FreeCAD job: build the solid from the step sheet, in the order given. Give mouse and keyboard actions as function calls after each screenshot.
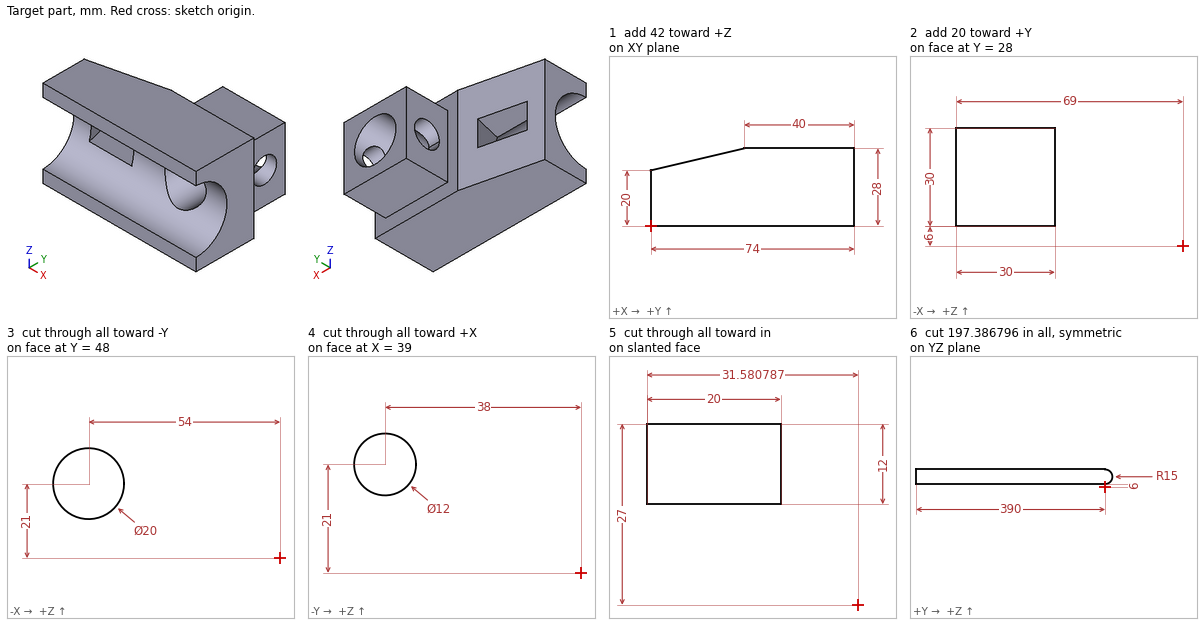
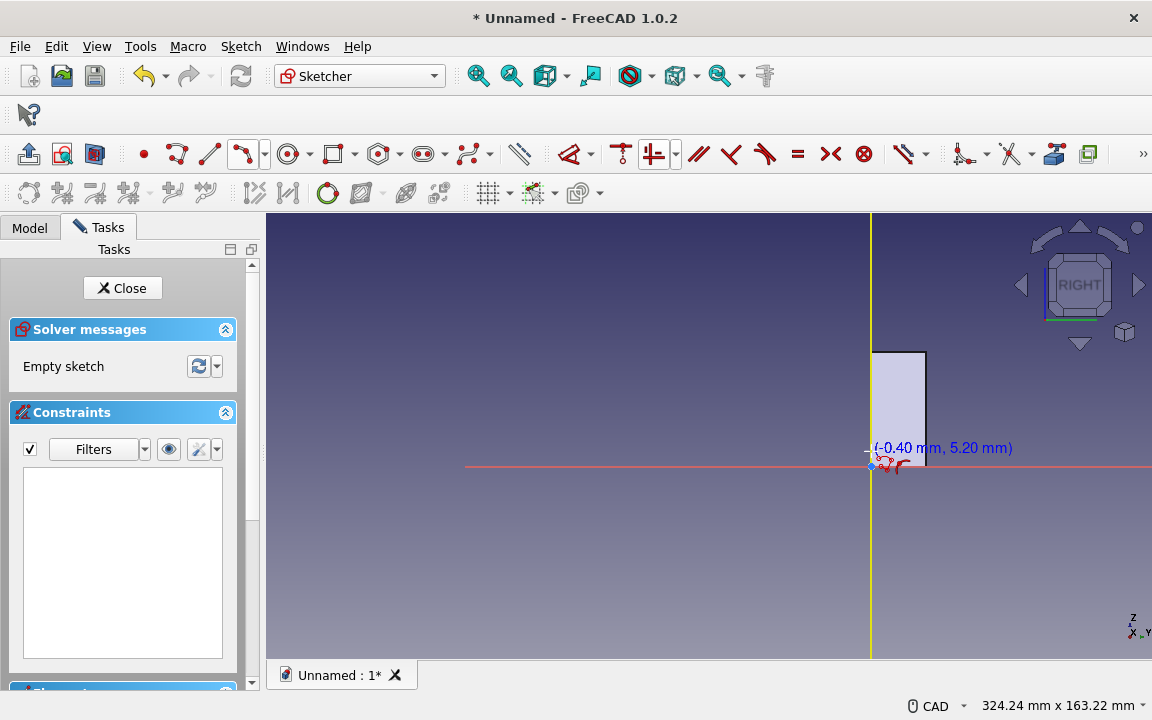
click(871, 450)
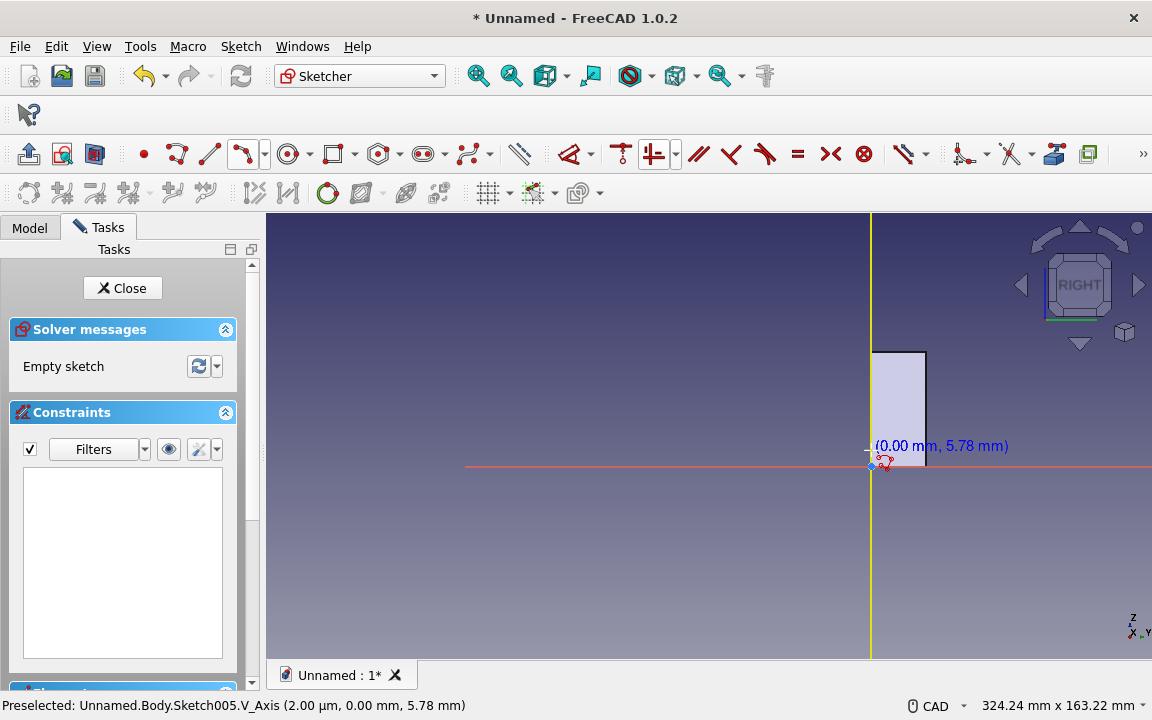
scroll(870, 451, down, 4)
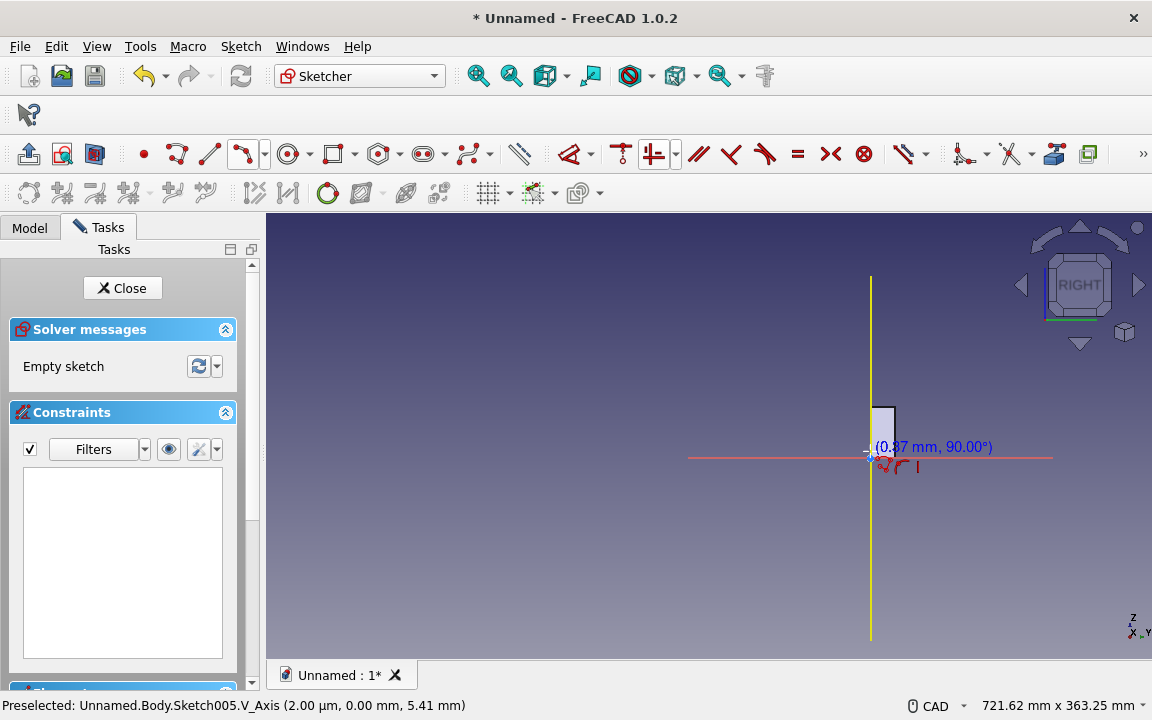
scroll(392, 451, up, 4)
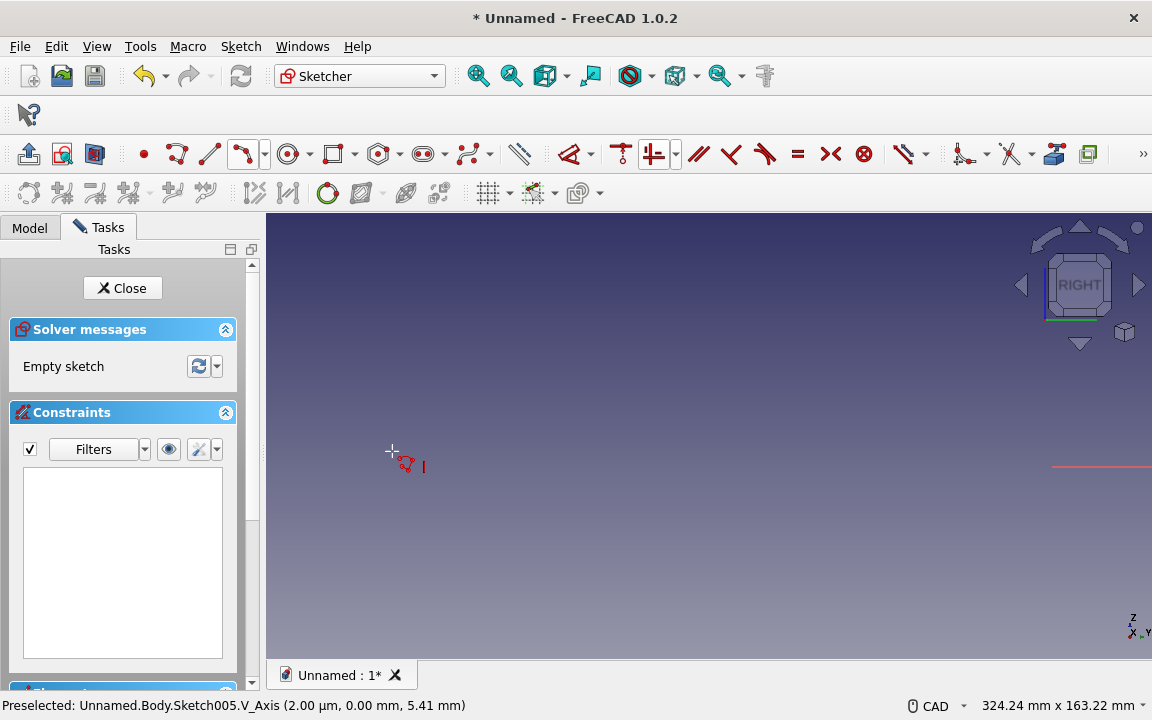
click(392, 450)
click(392, 368)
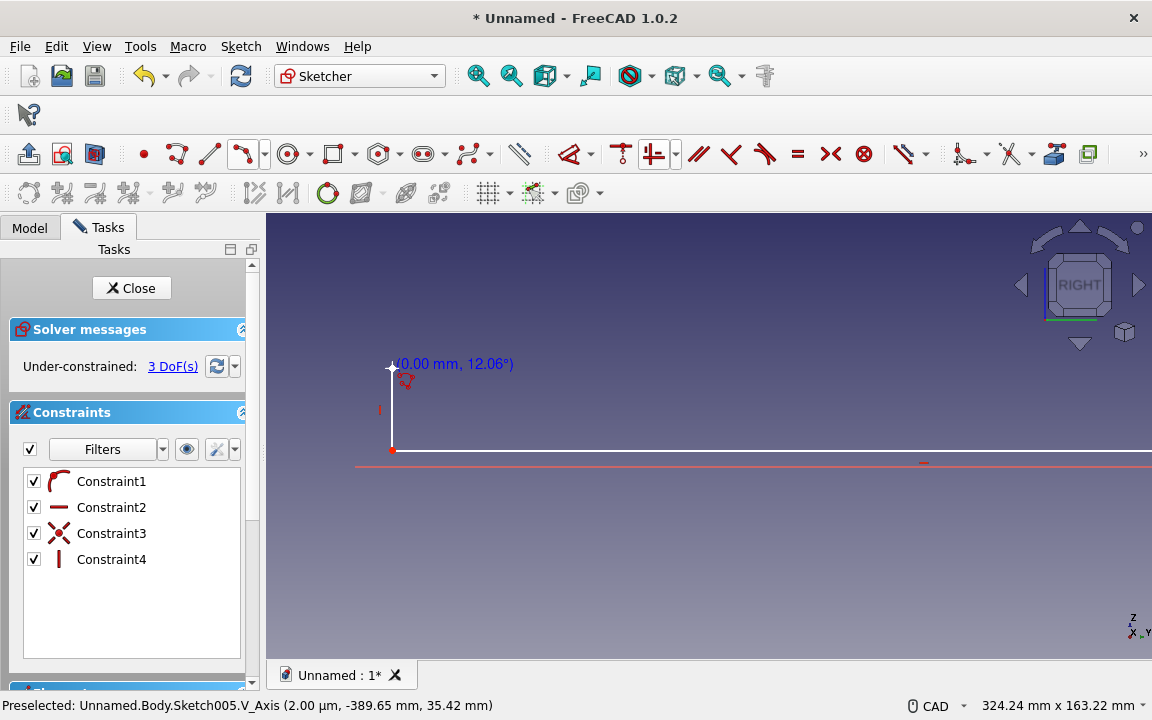
scroll(392, 451, down, 4)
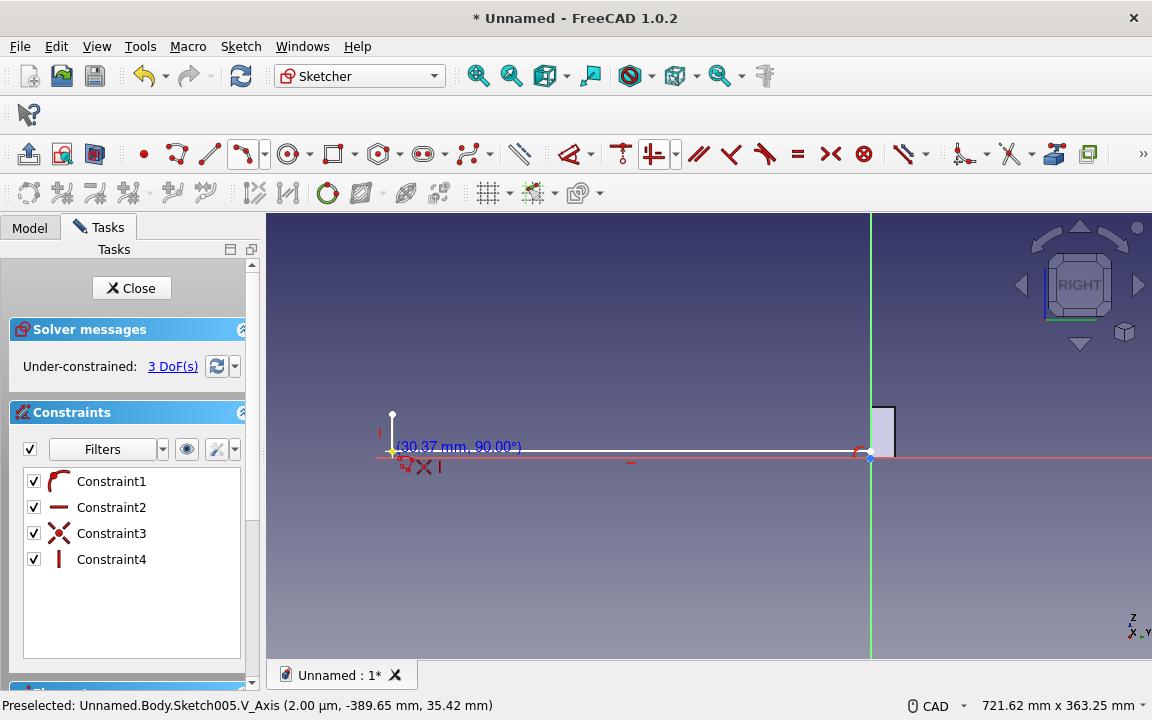
click(871, 414)
right_click(871, 414)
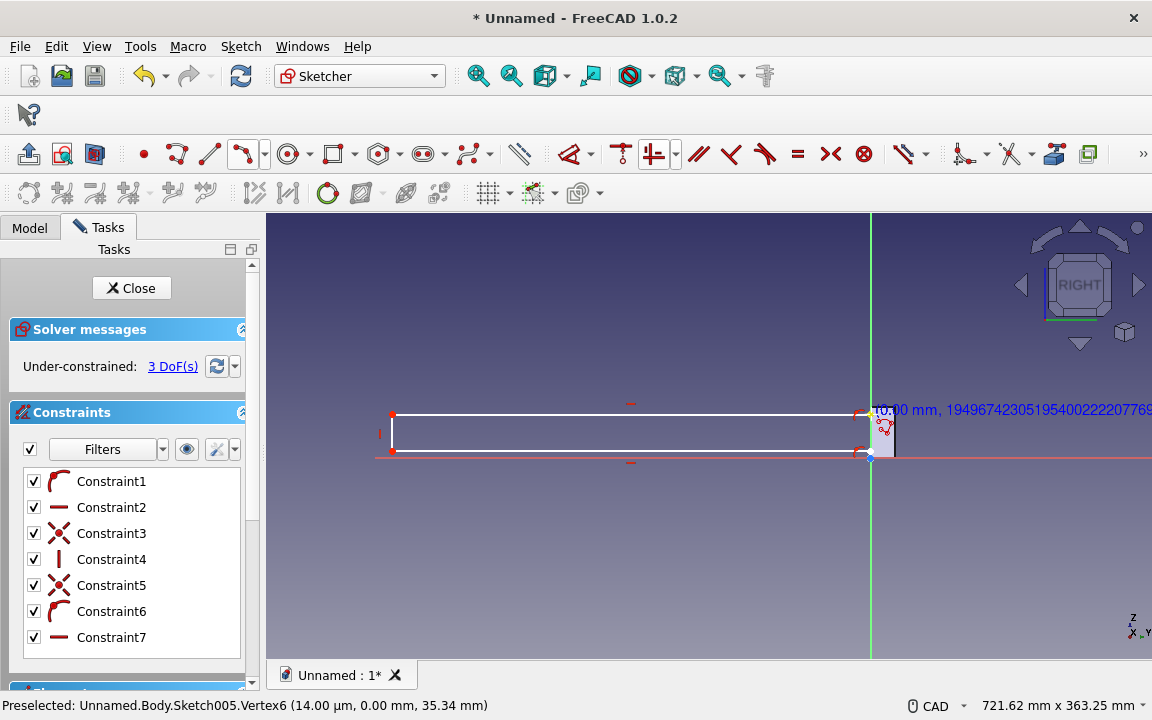
click(242, 154)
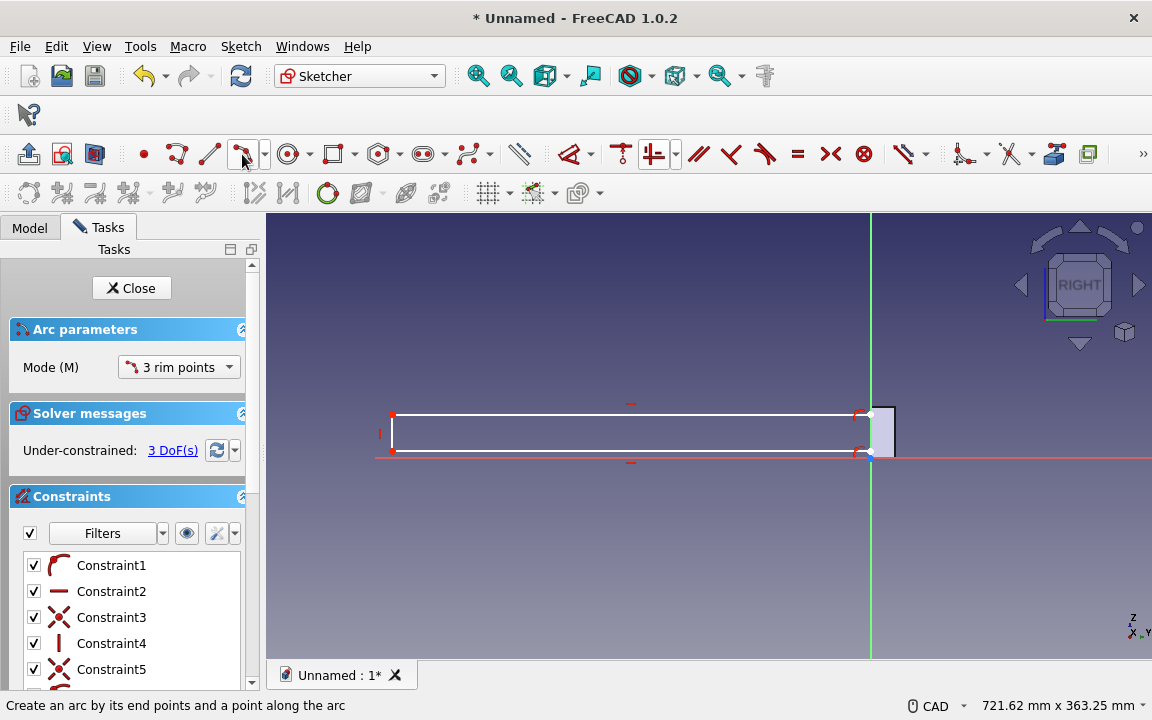
click(871, 415)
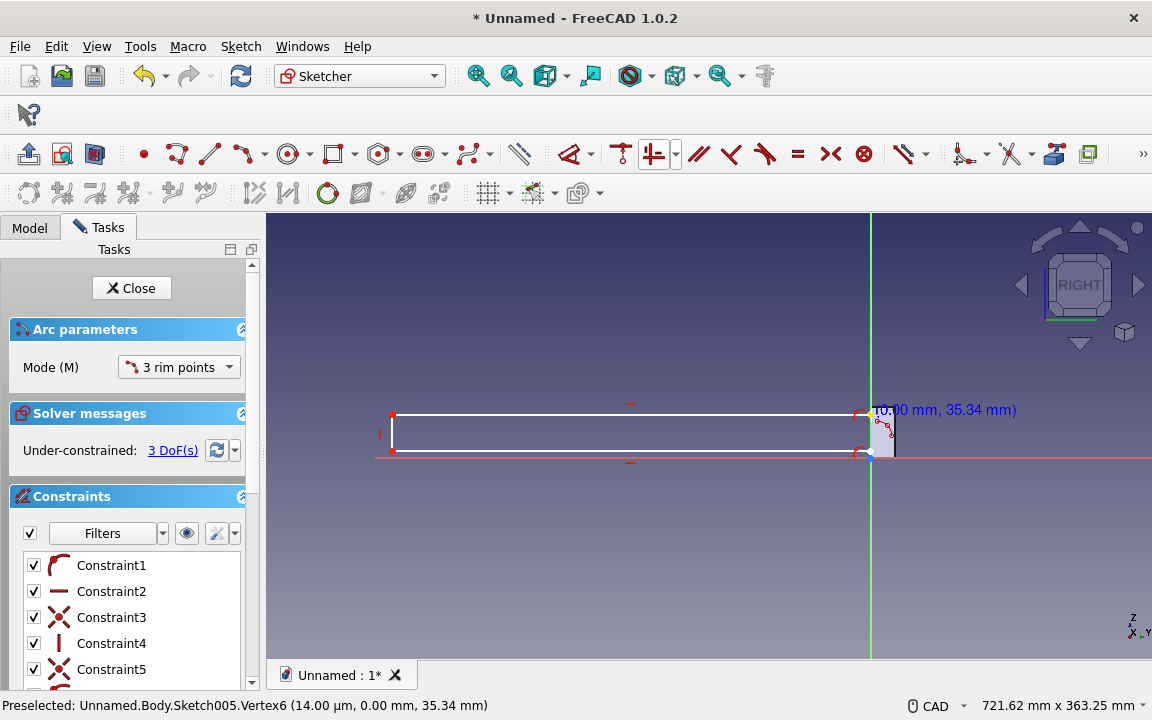
scroll(871, 451, up, 4)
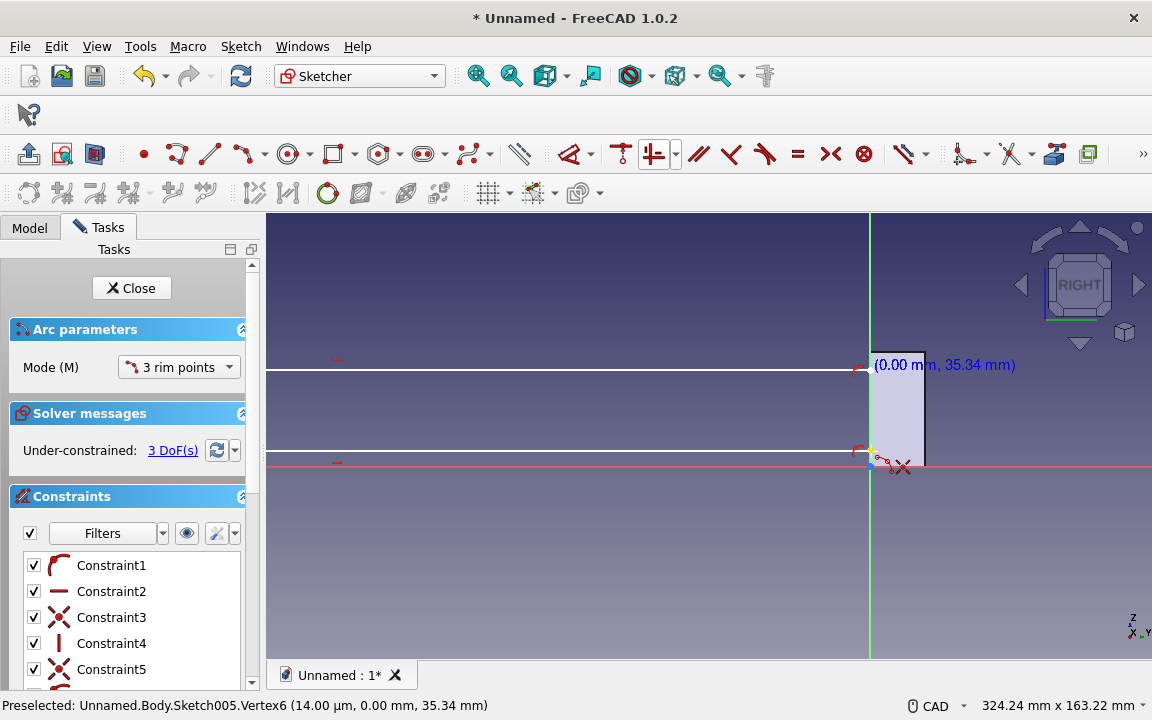
click(870, 451)
click(911, 409)
key(Escape)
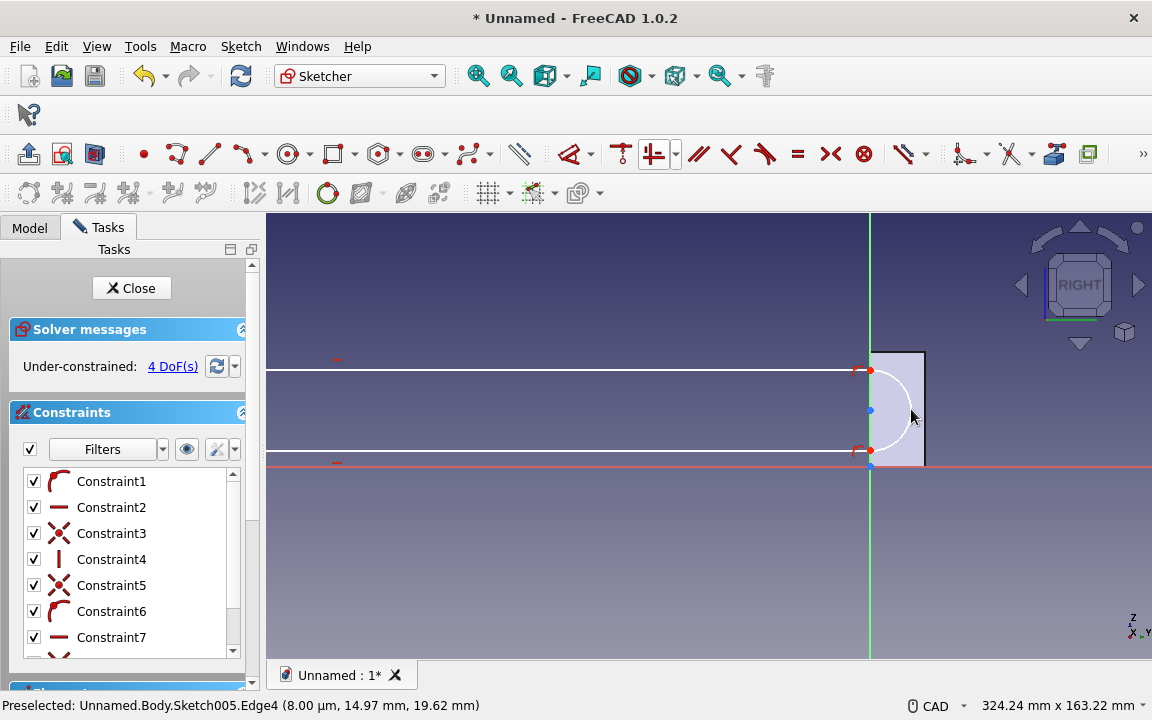
click(550, 451)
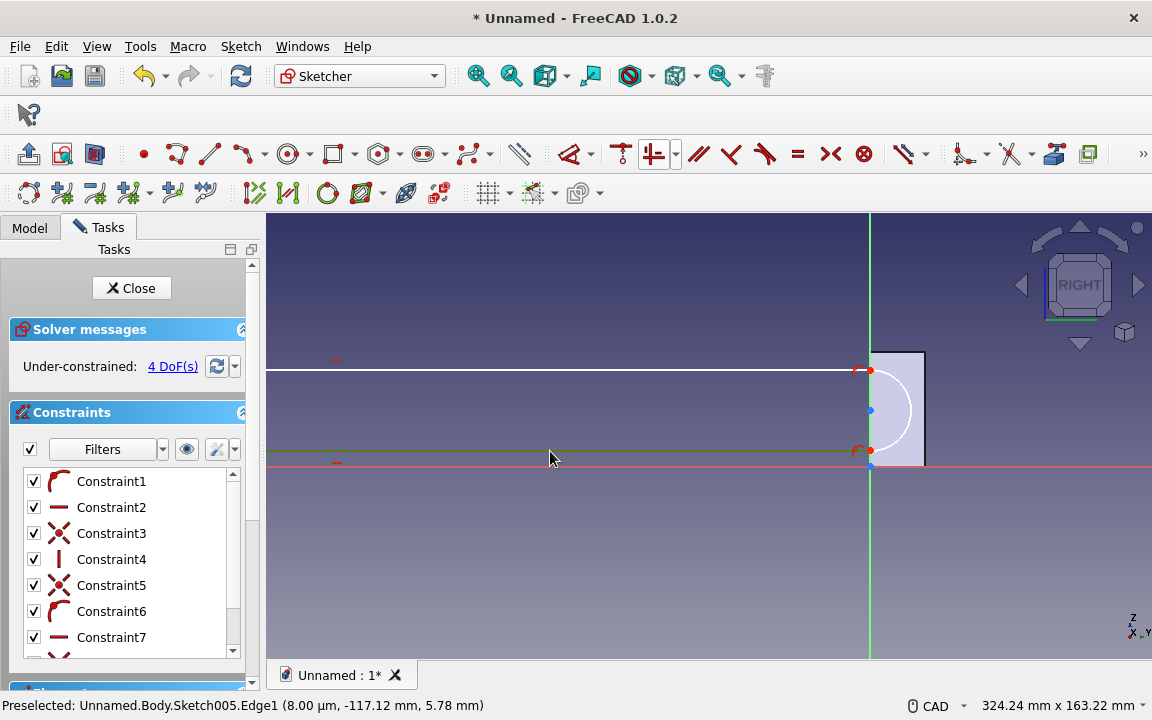
click(903, 435)